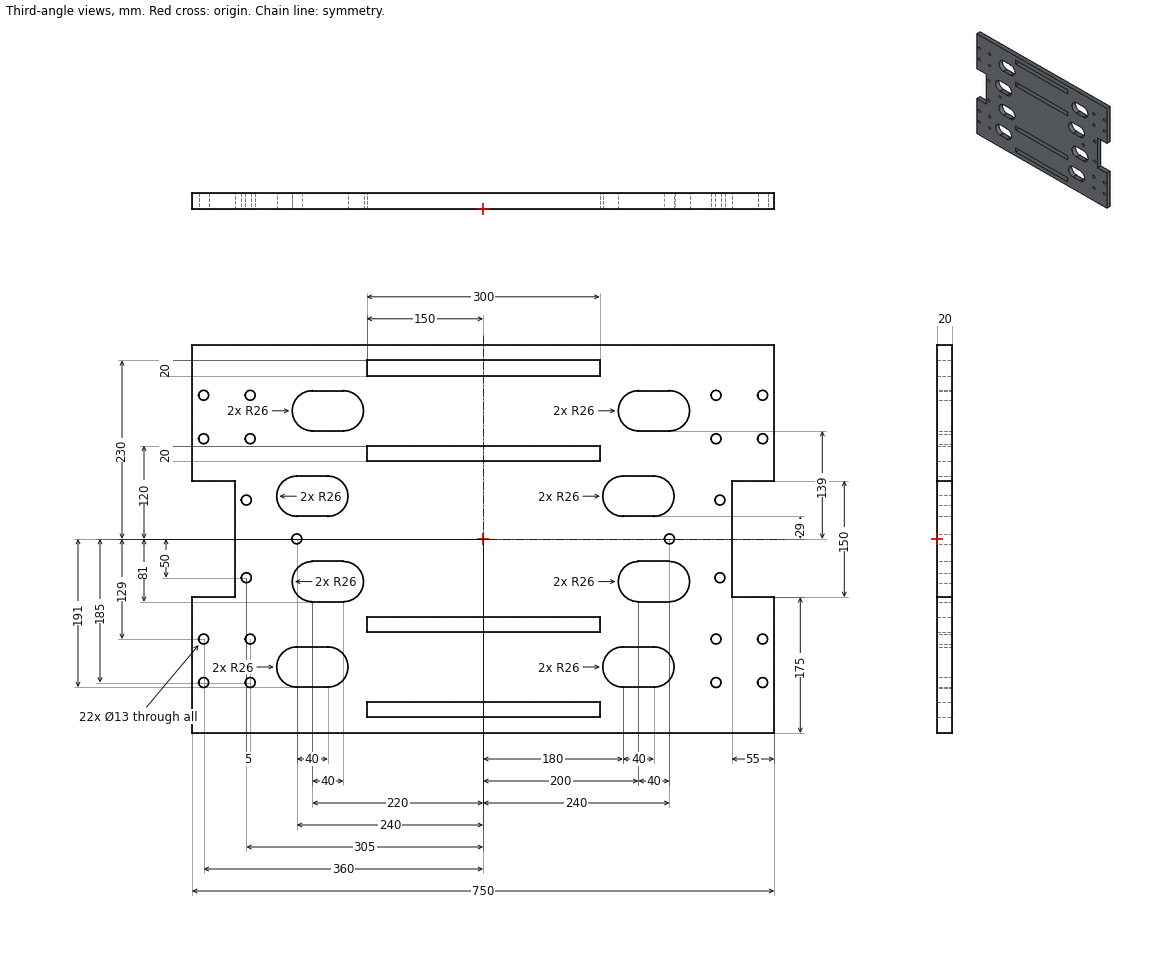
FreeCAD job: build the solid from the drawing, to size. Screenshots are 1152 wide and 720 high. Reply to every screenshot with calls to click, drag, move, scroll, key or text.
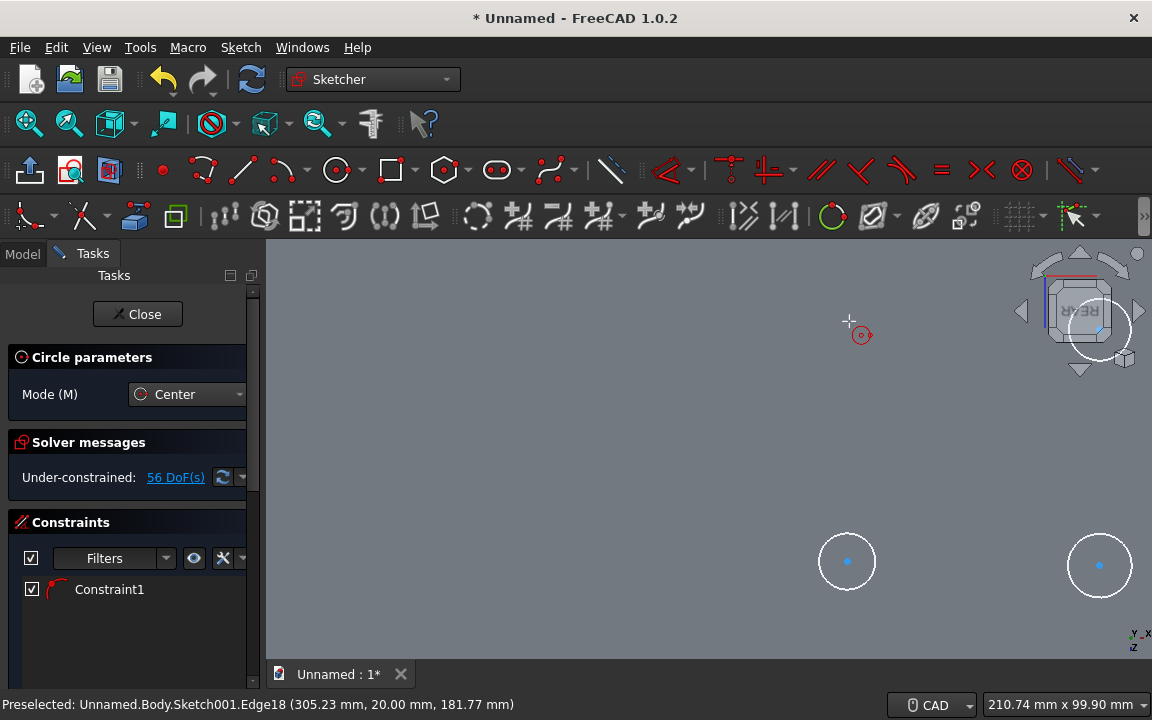
scroll(849, 320, down, 9)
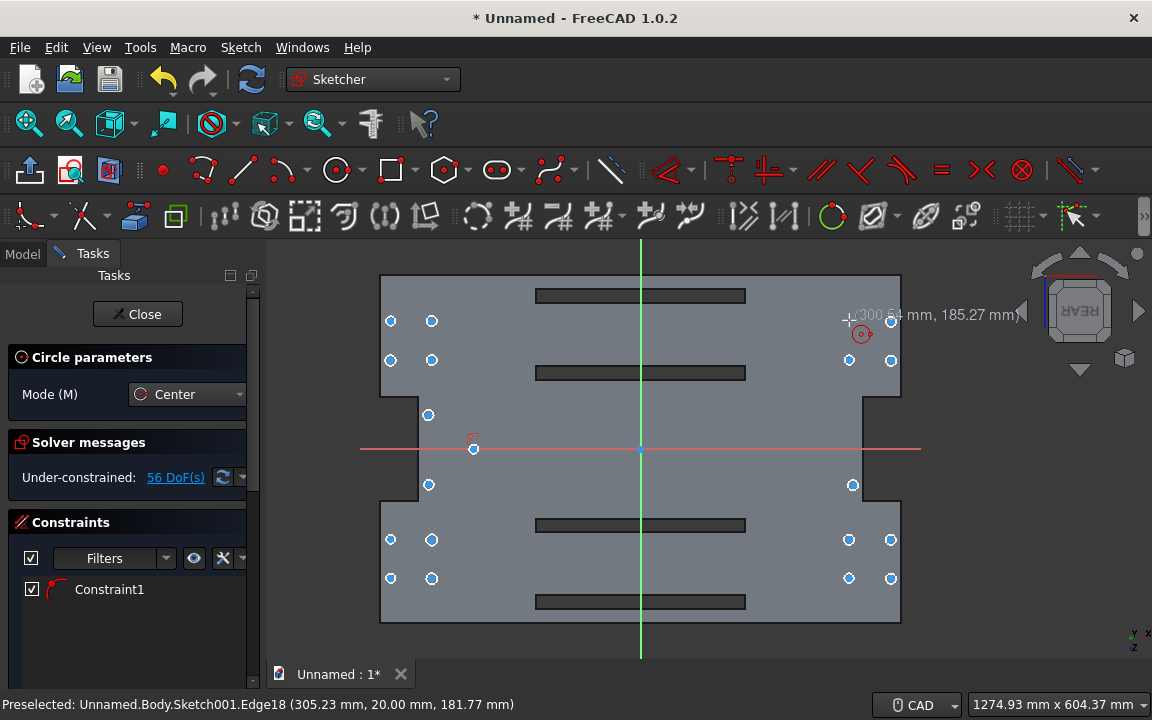
click(849, 321)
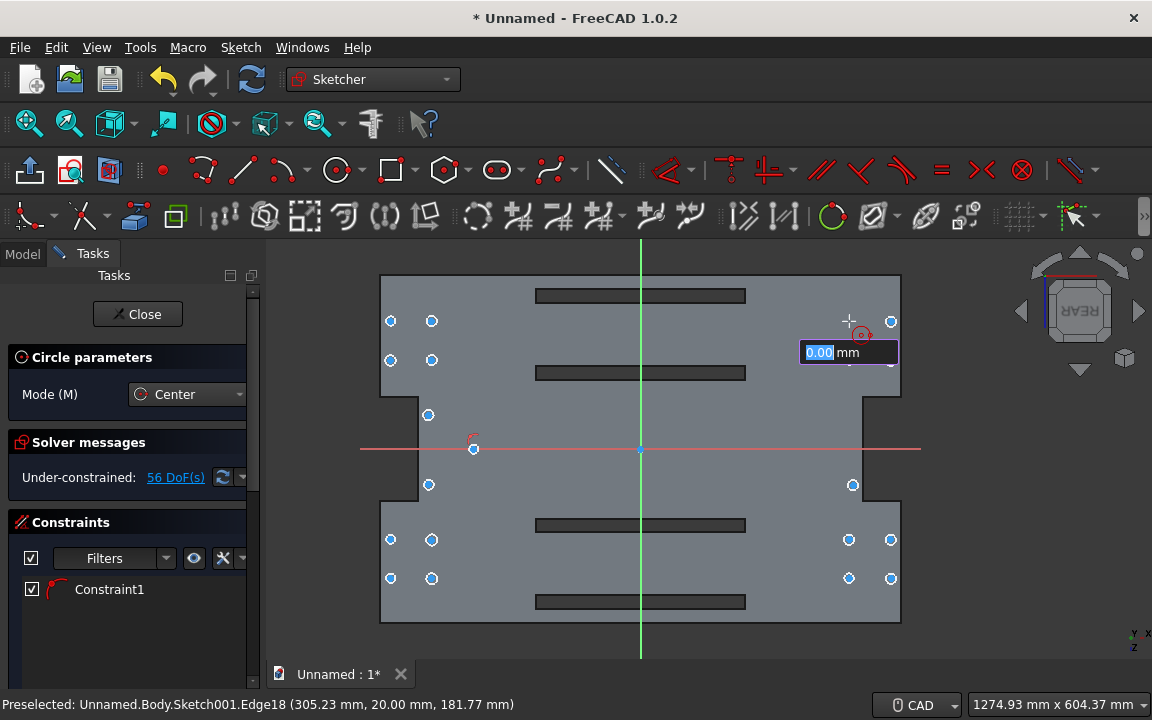
scroll(852, 317, up, 7)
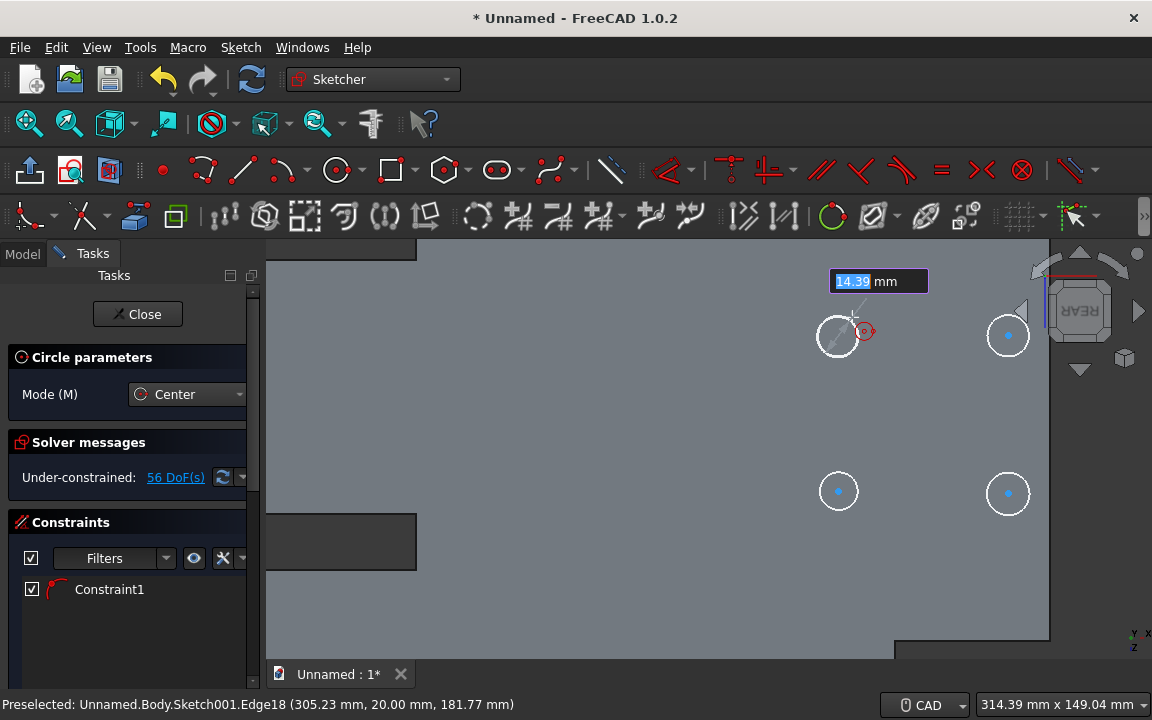
click(851, 318)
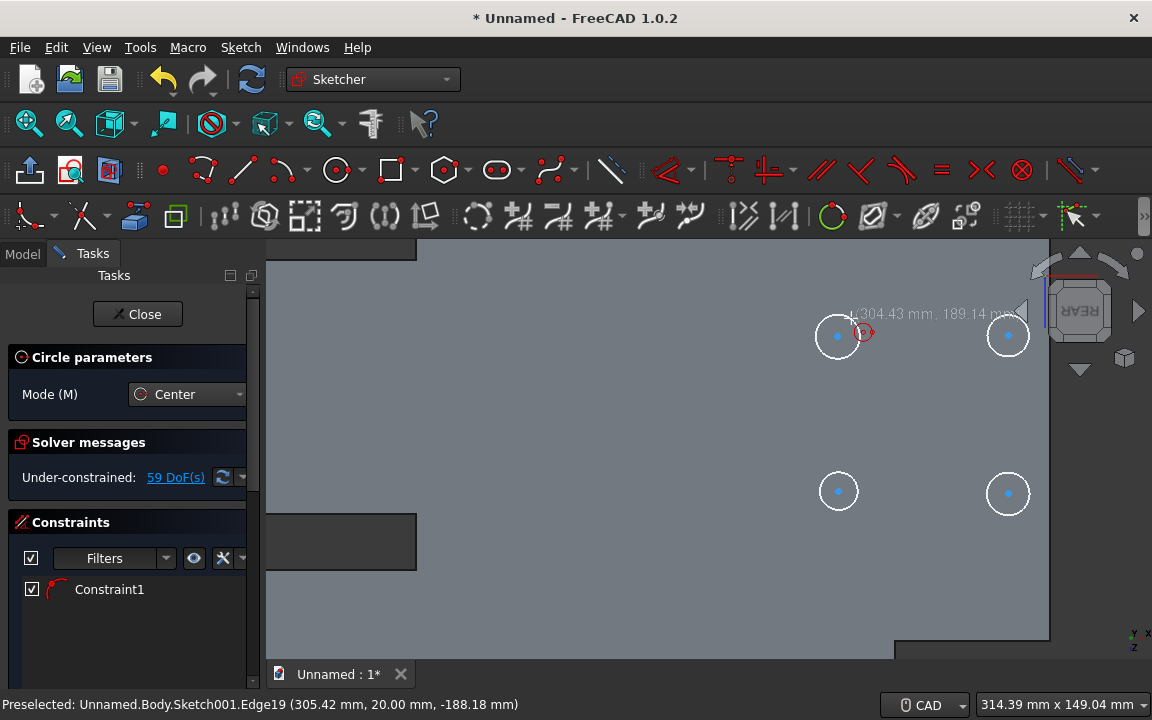
scroll(852, 317, down, 7)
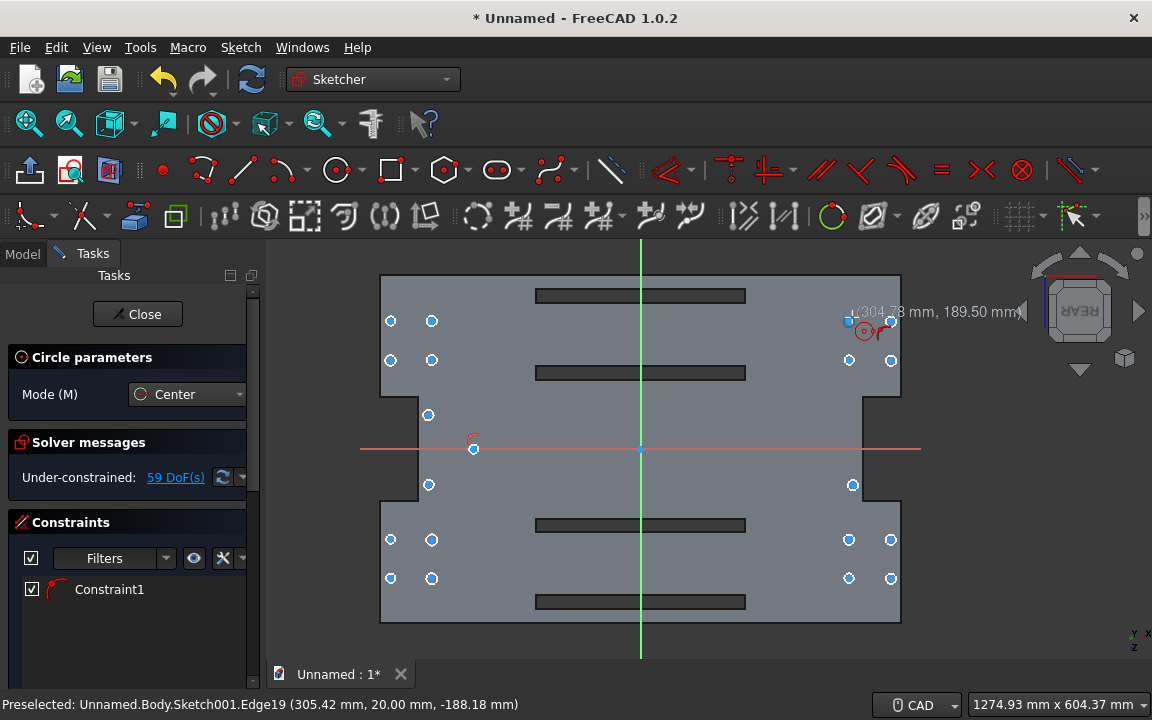
scroll(807, 449, up, 9)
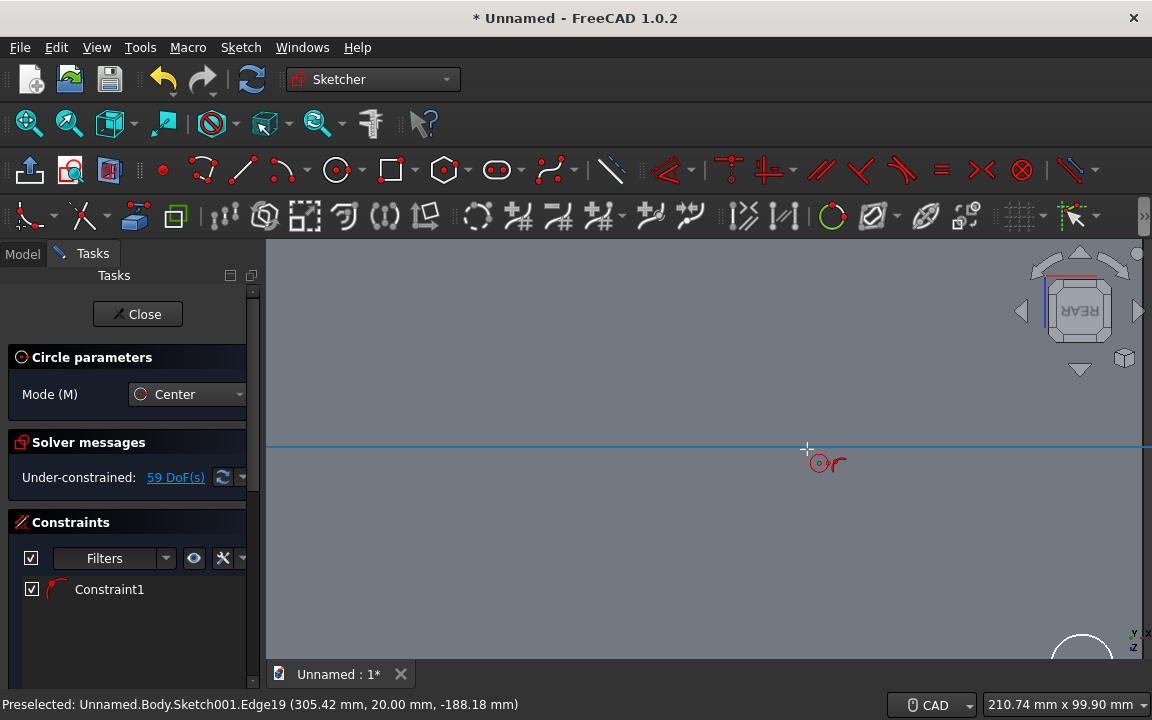
scroll(807, 449, down, 9)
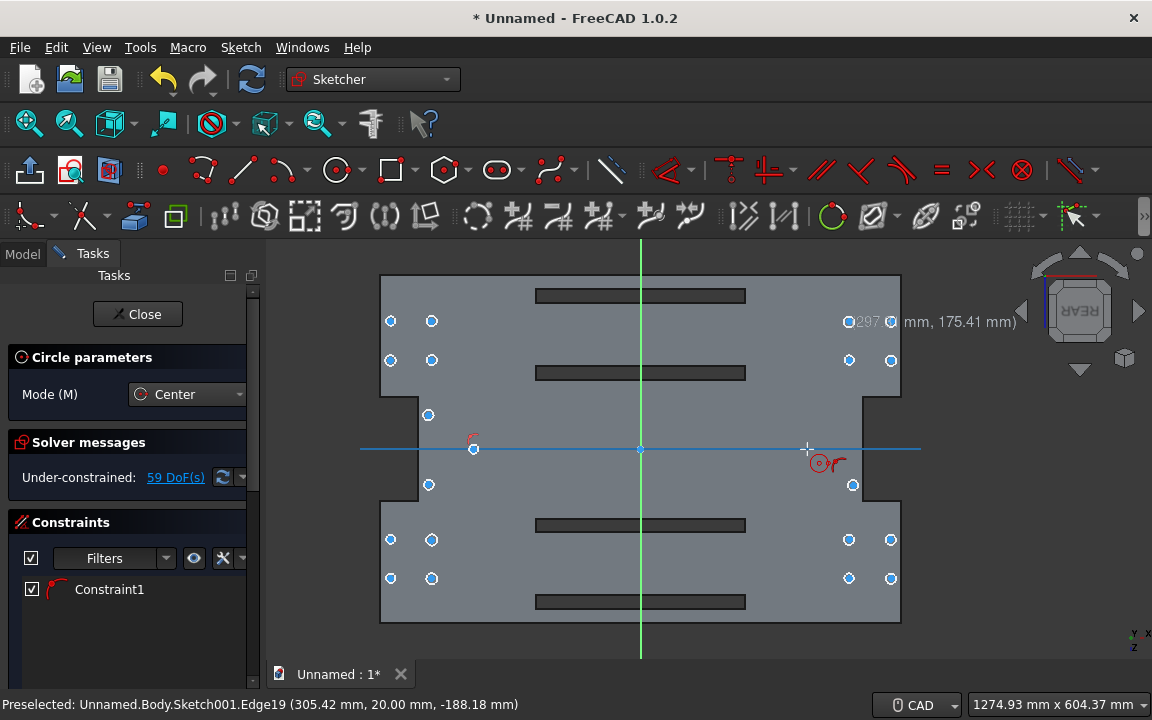
click(807, 449)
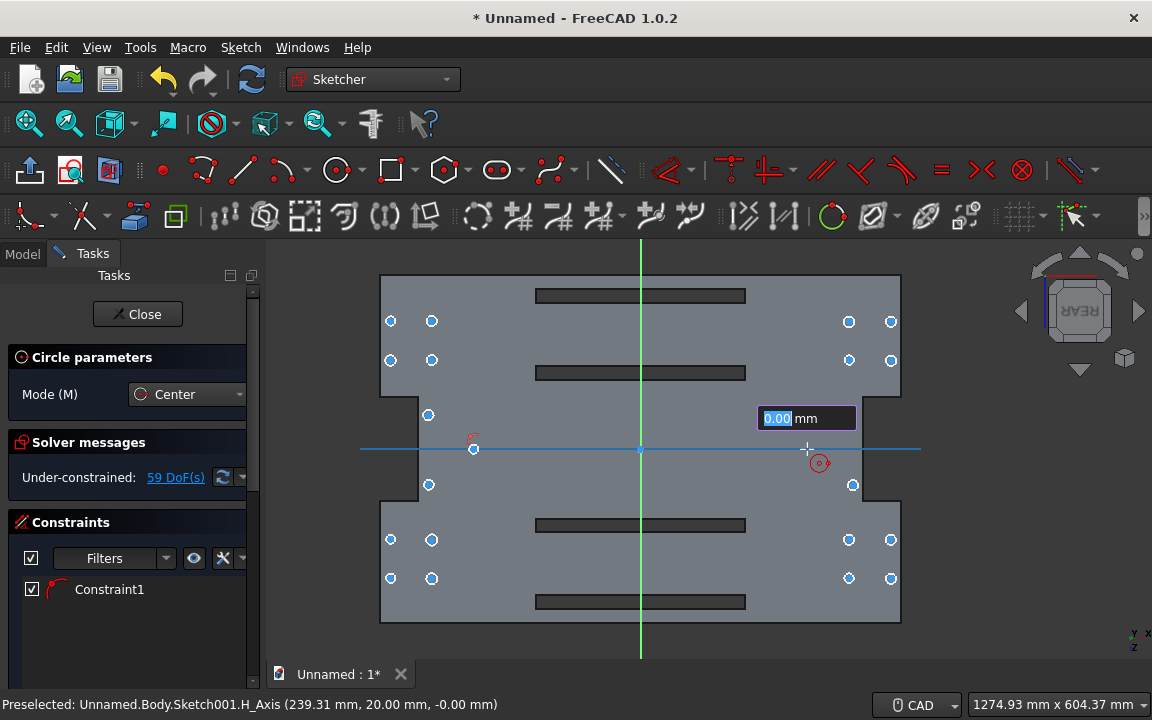
scroll(806, 453, up, 7)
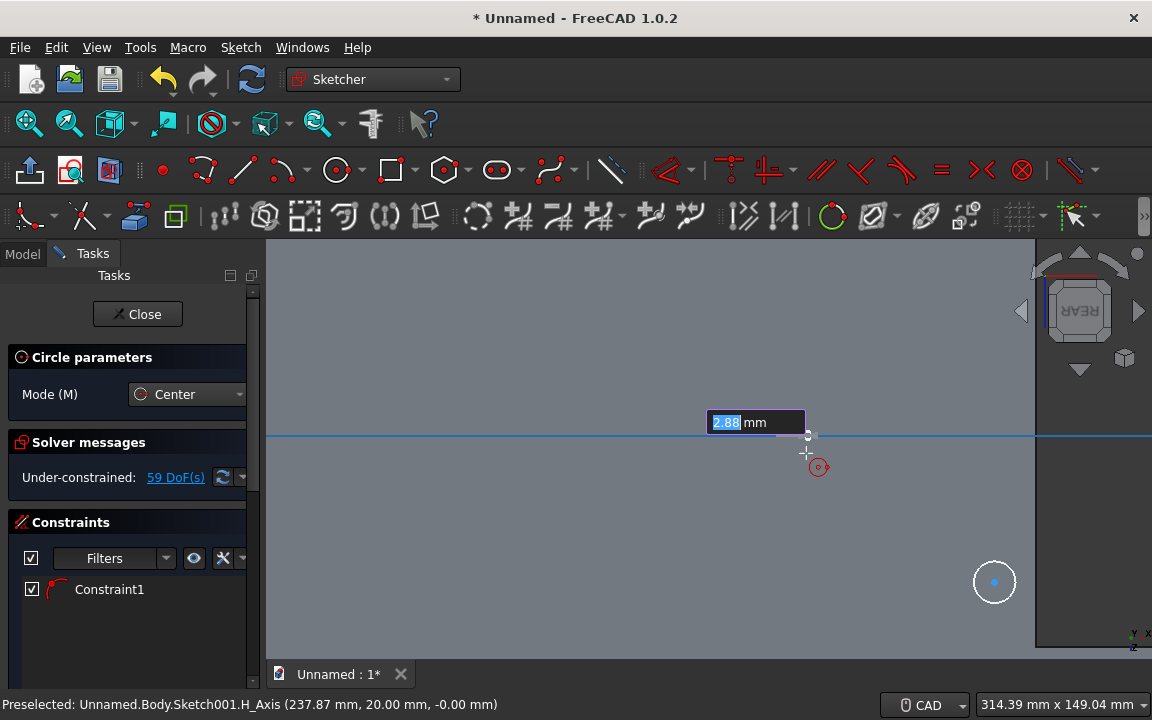
click(804, 453)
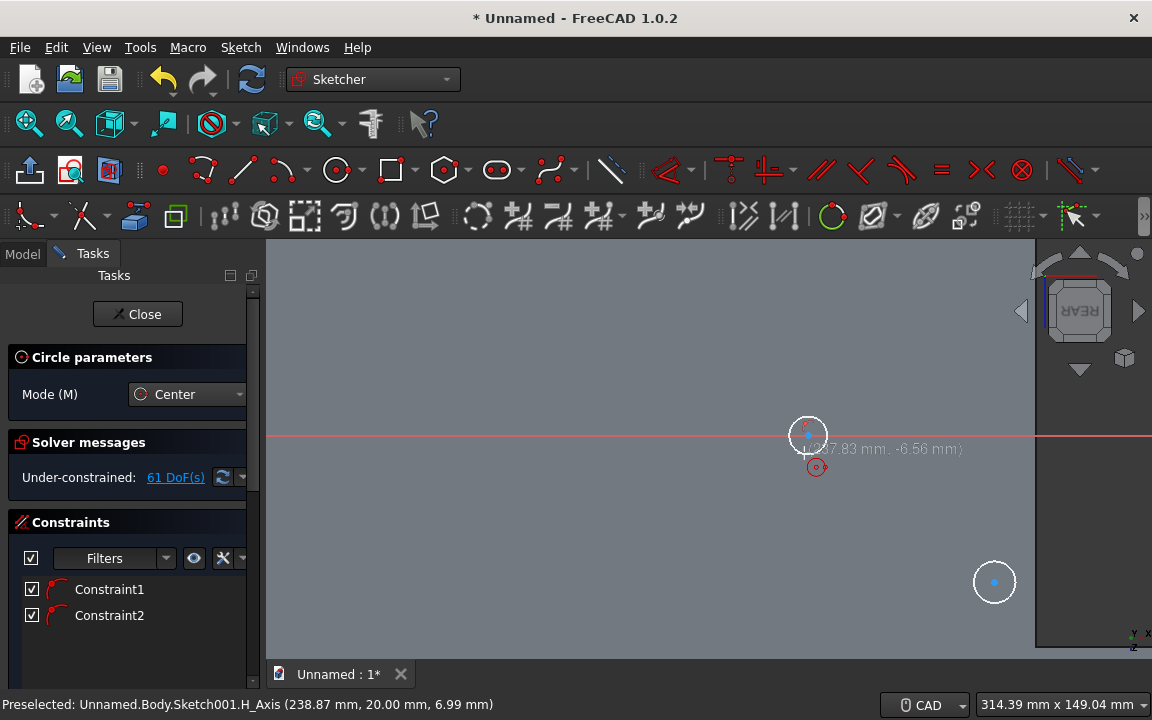
scroll(806, 453, down, 7)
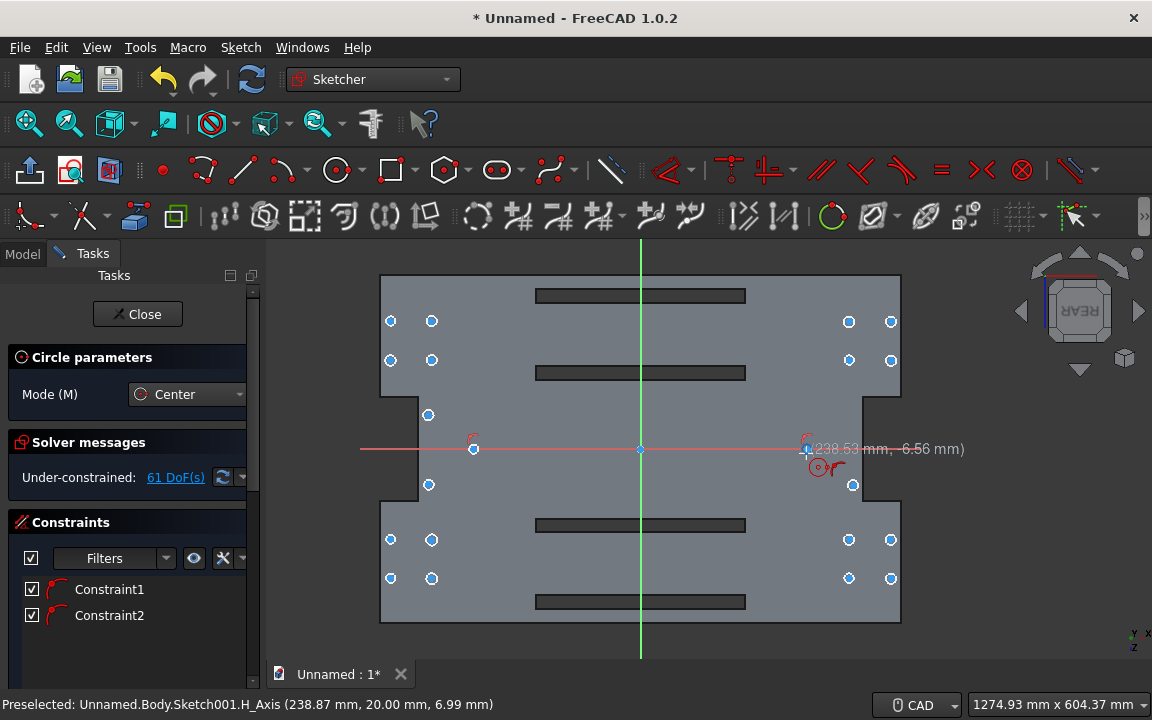
scroll(853, 414, up, 9)